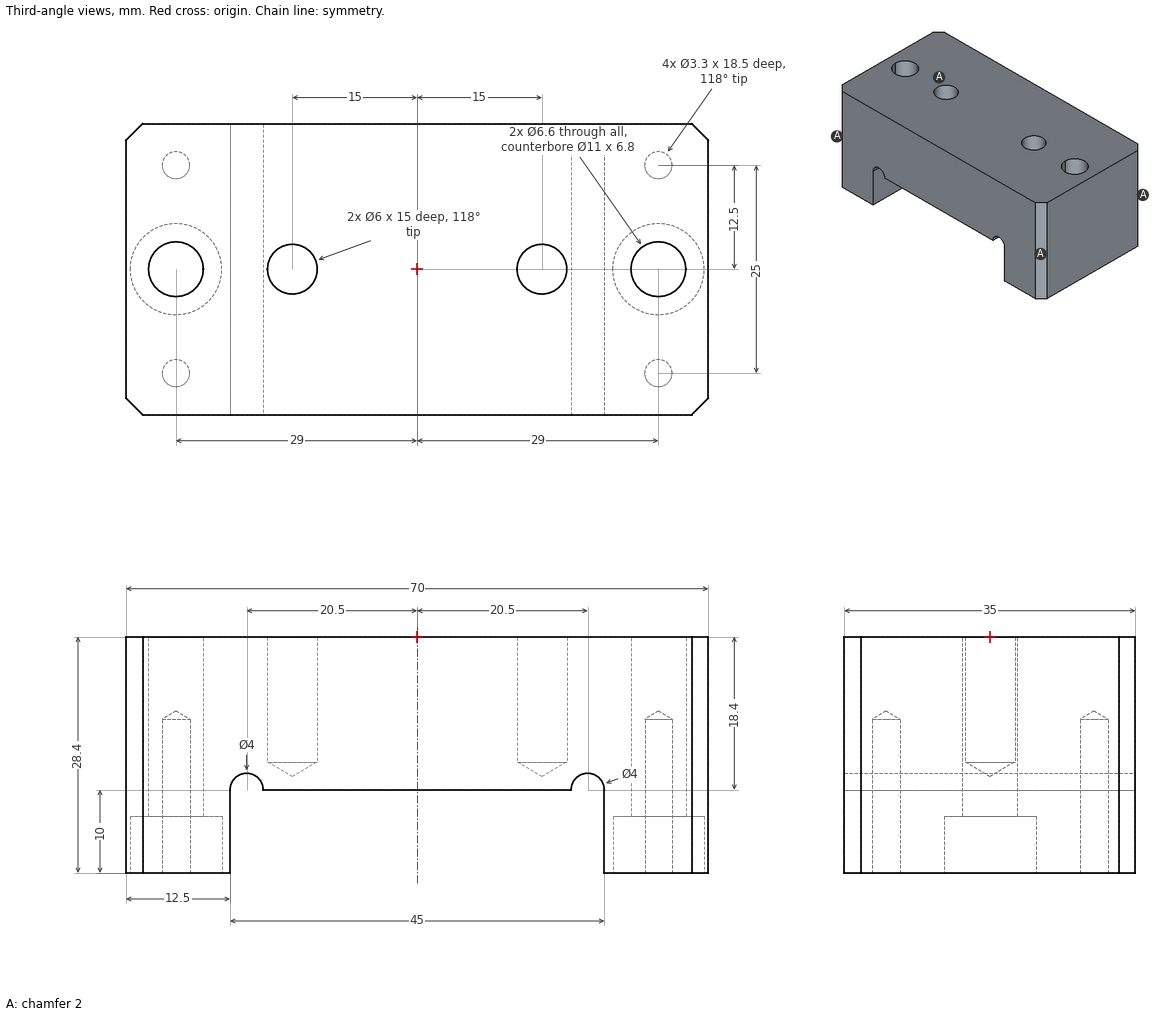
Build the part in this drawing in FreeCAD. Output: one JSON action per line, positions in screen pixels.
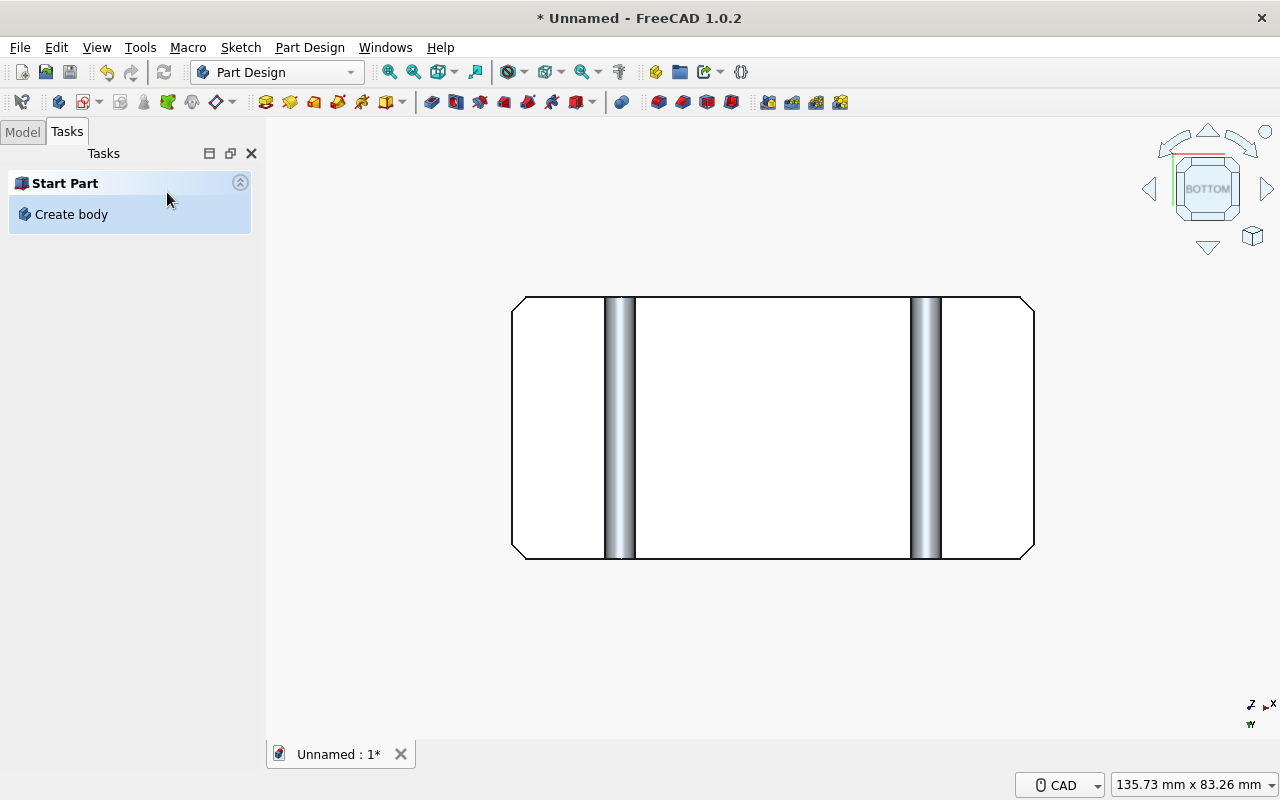
{"action": "left_click", "coordinate": [558, 502]}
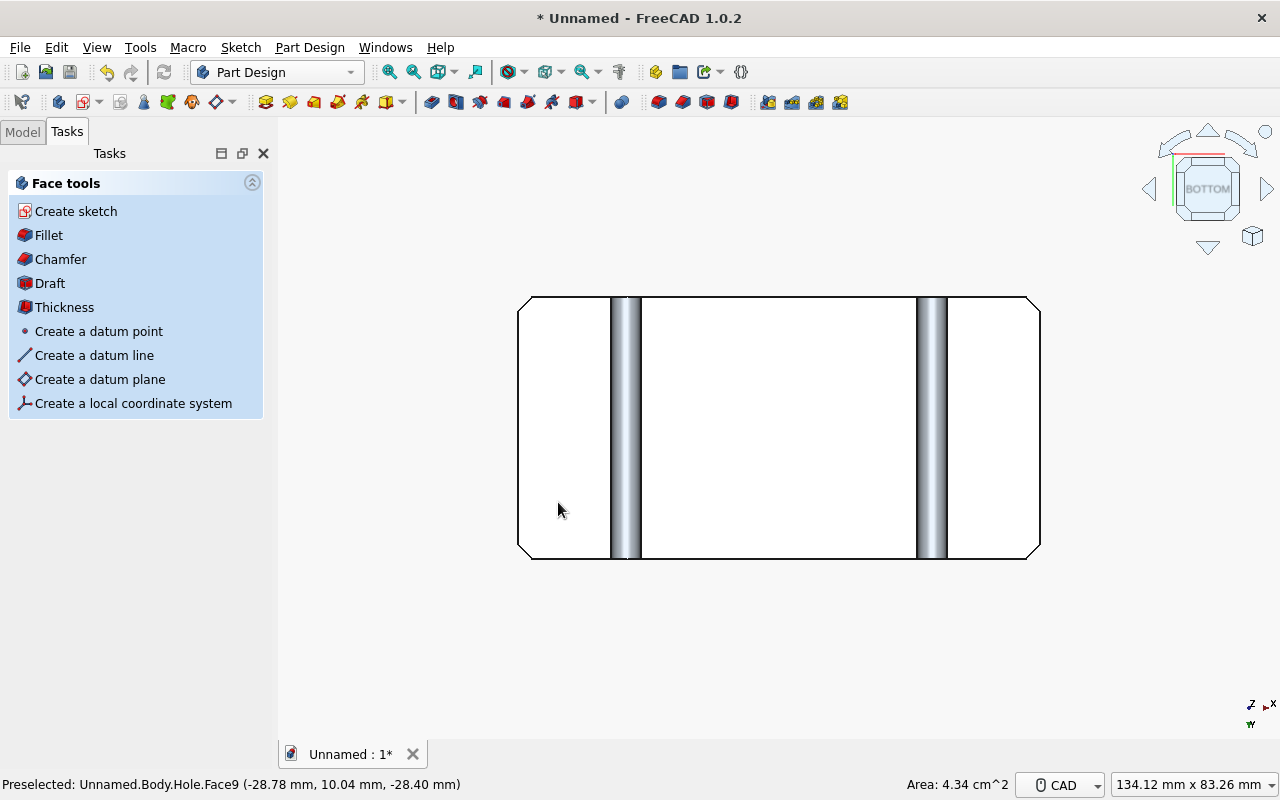
{"action": "left_click", "coordinate": [84, 102]}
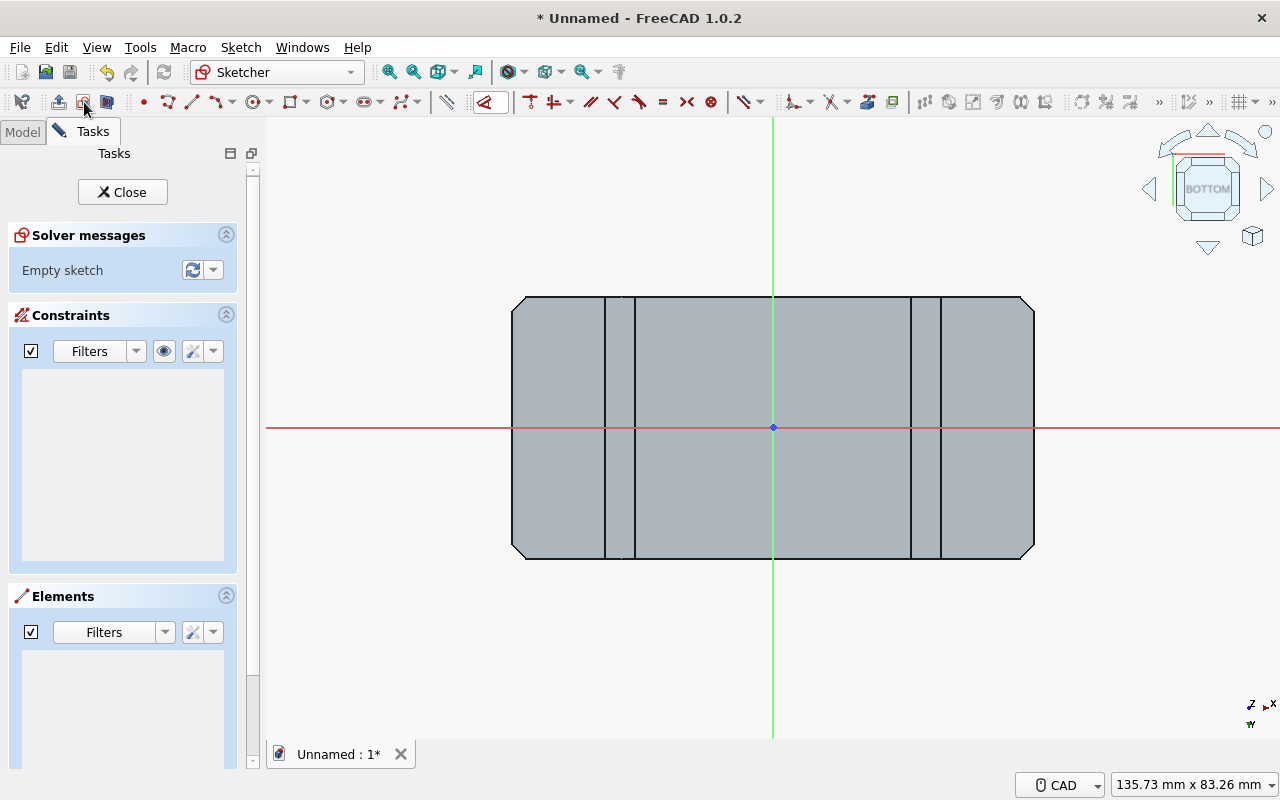
{"action": "left_click", "coordinate": [254, 102]}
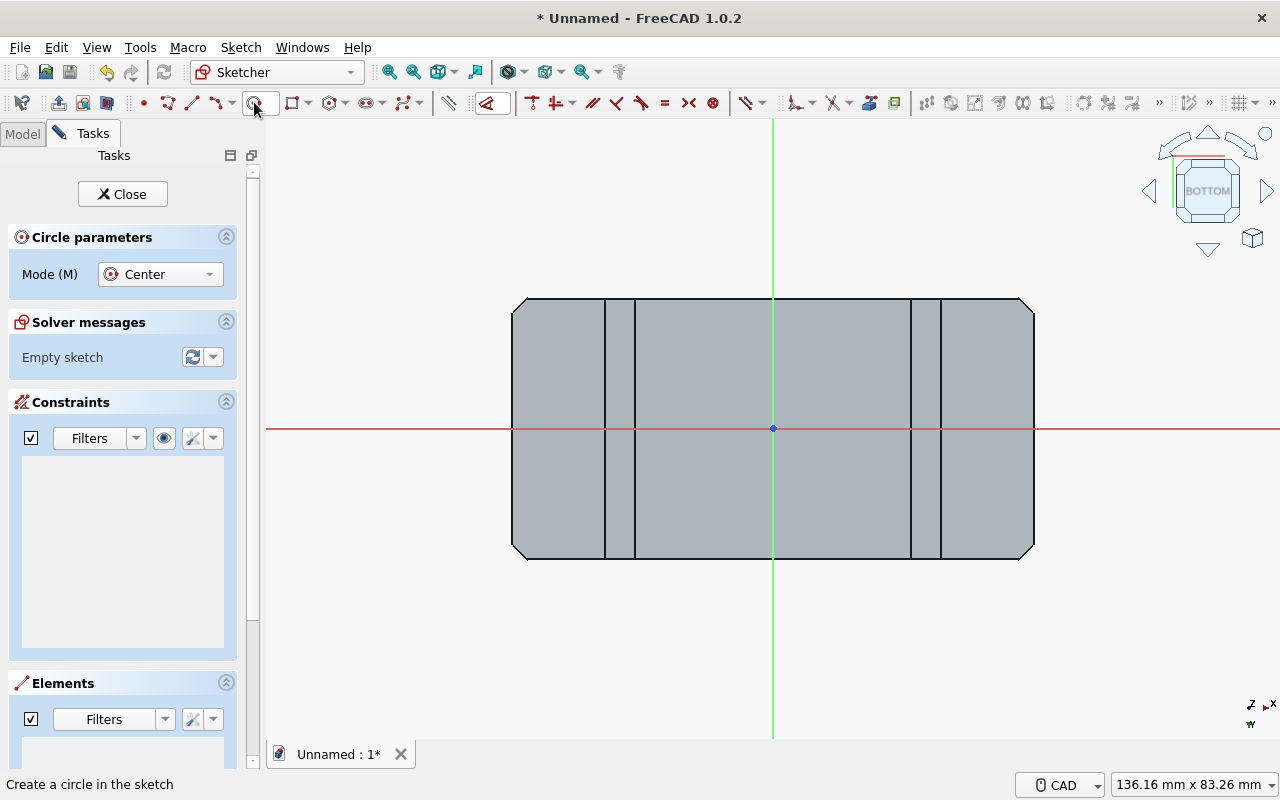
{"action": "left_click", "coordinate": [989, 429]}
{"action": "left_click", "coordinate": [1006, 412]}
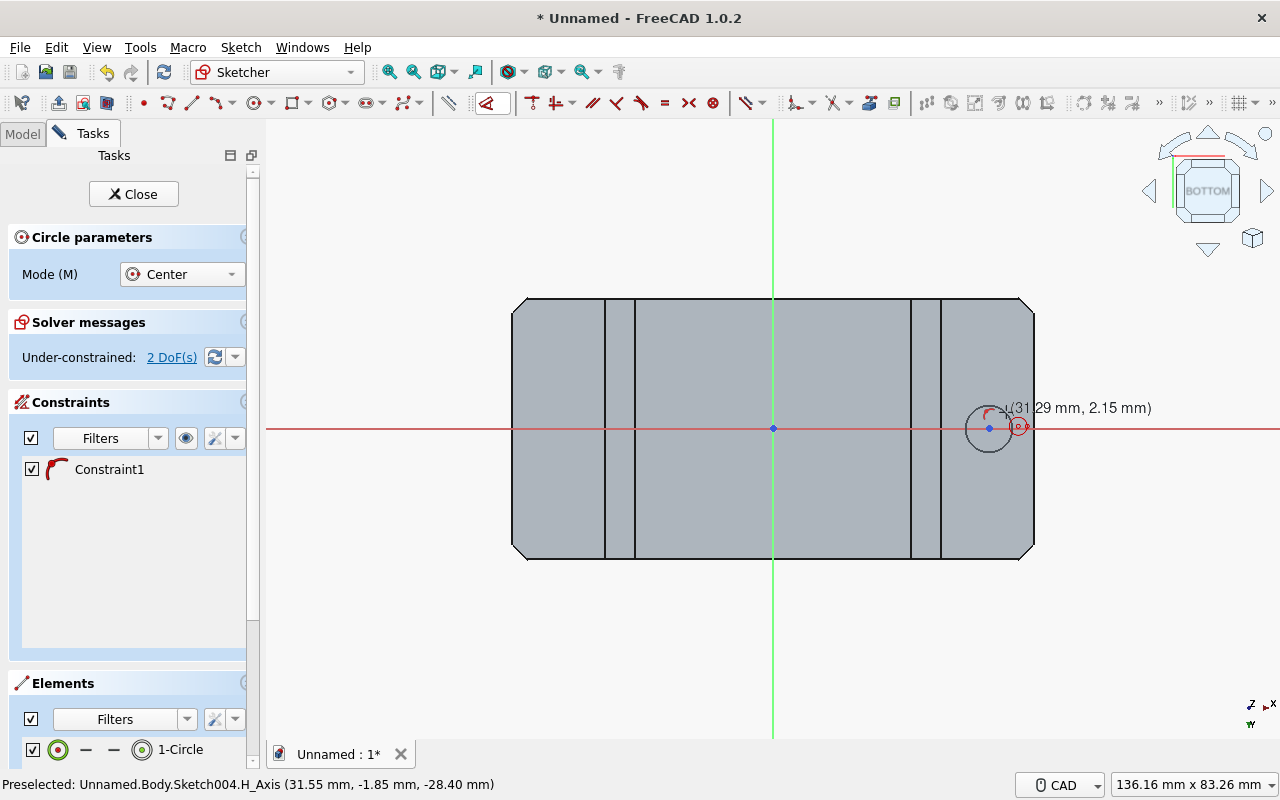
{"action": "left_click", "coordinate": [557, 429]}
{"action": "left_click", "coordinate": [574, 412]}
{"action": "key", "text": "Escape"}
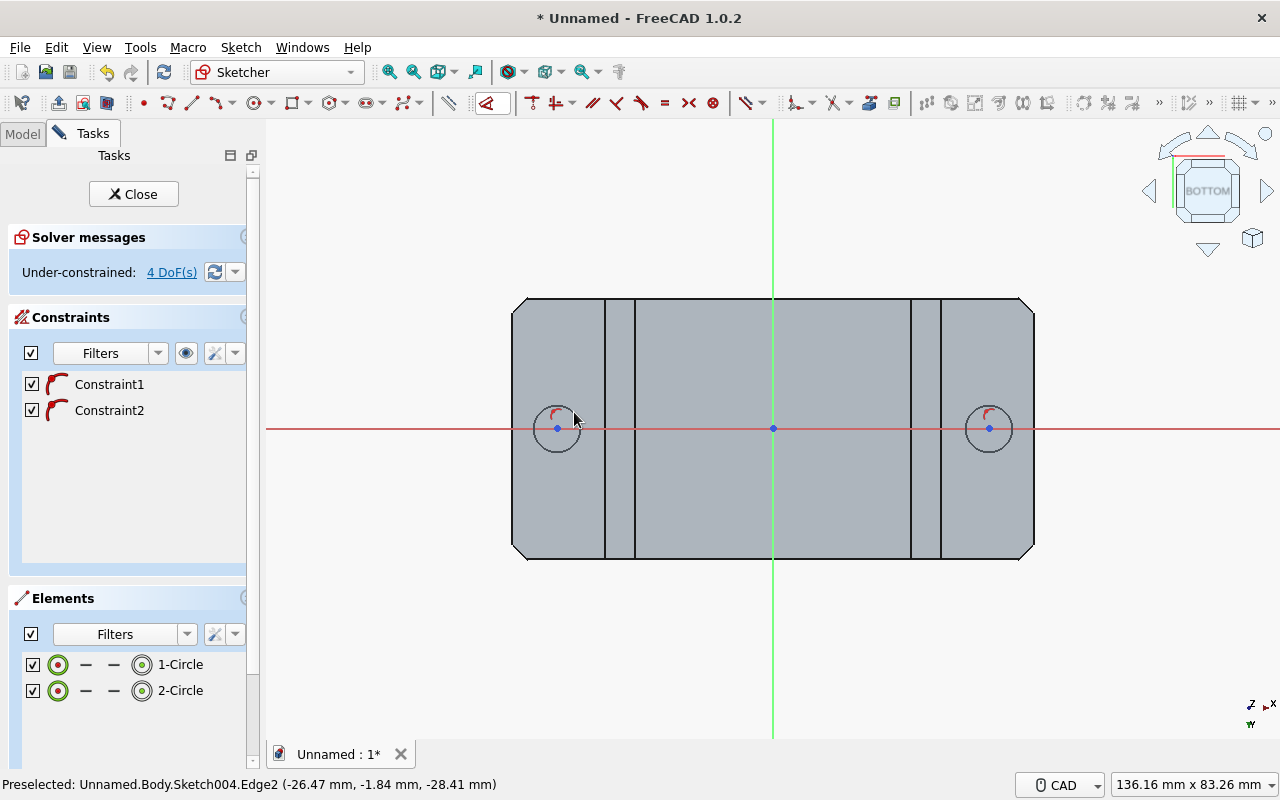
{"action": "left_click", "coordinate": [1005, 412]}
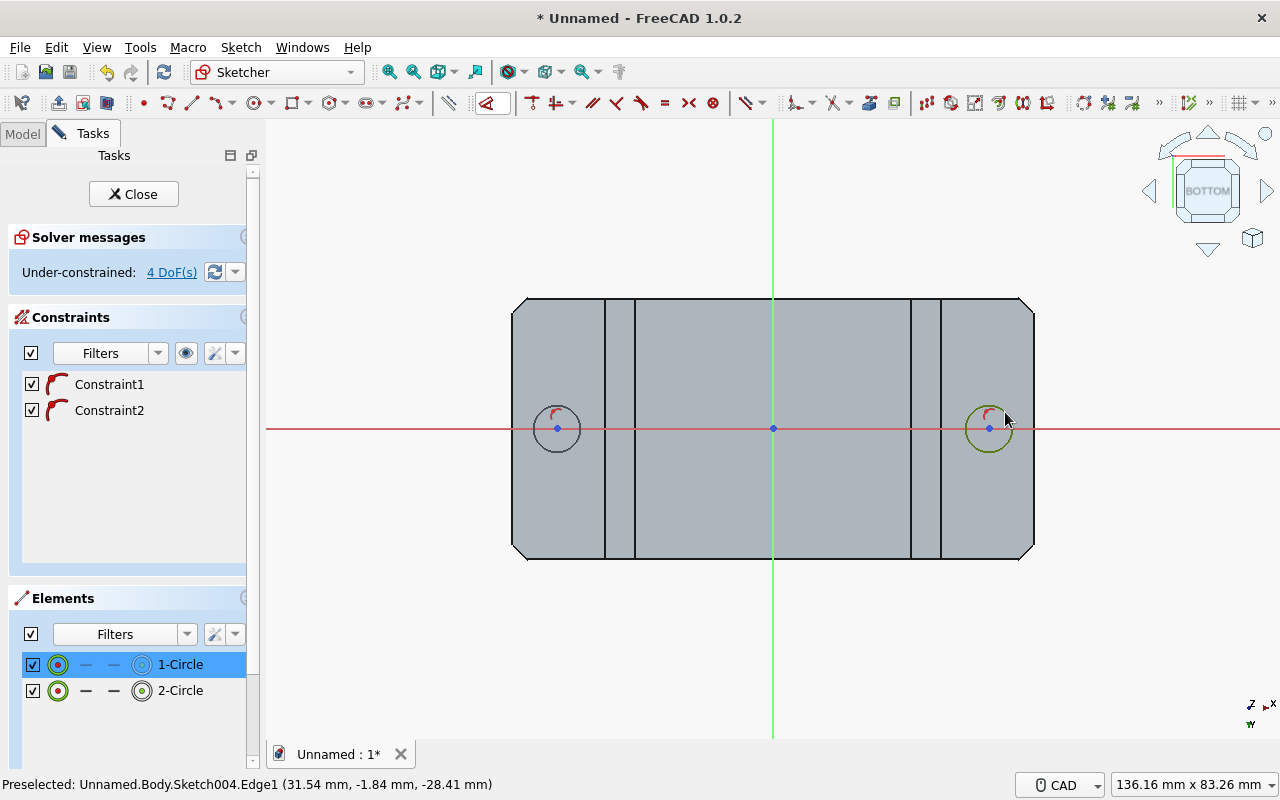
{"action": "left_click", "coordinate": [573, 412]}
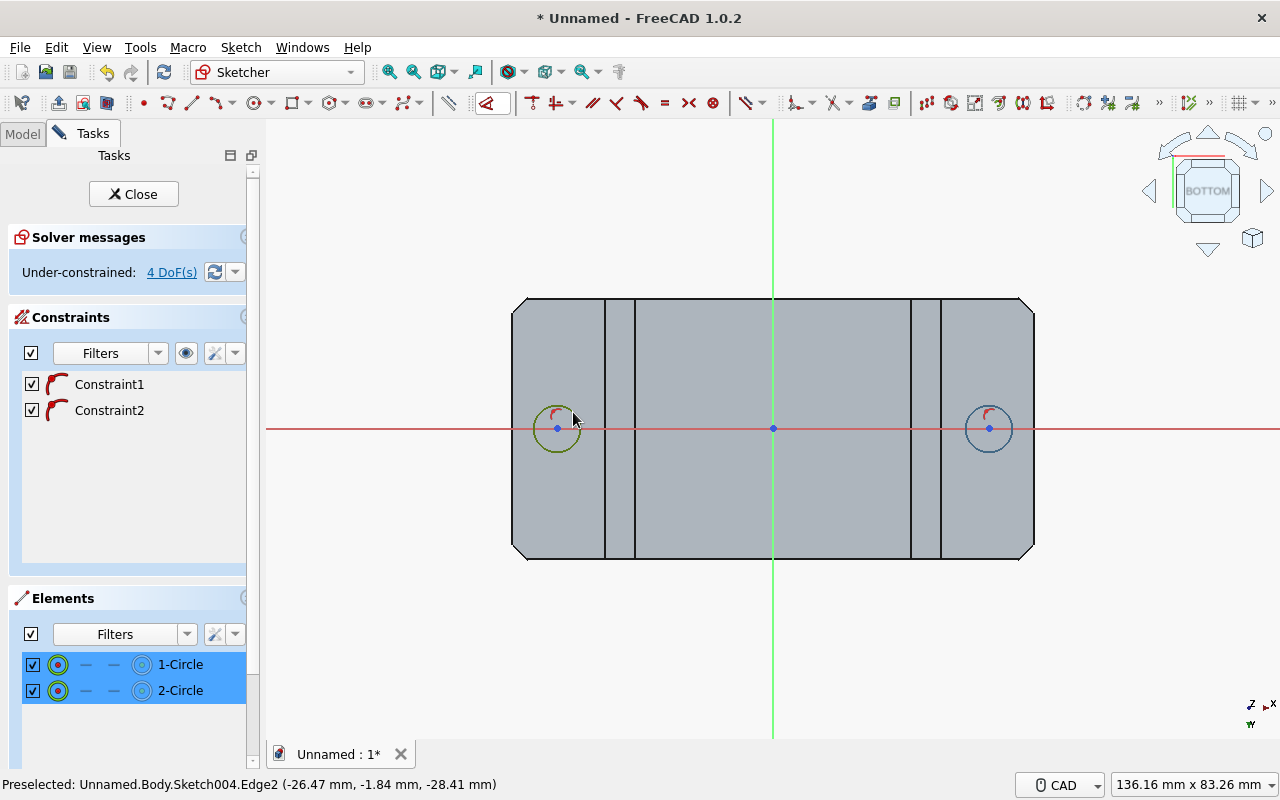
{"action": "left_click", "coordinate": [666, 104]}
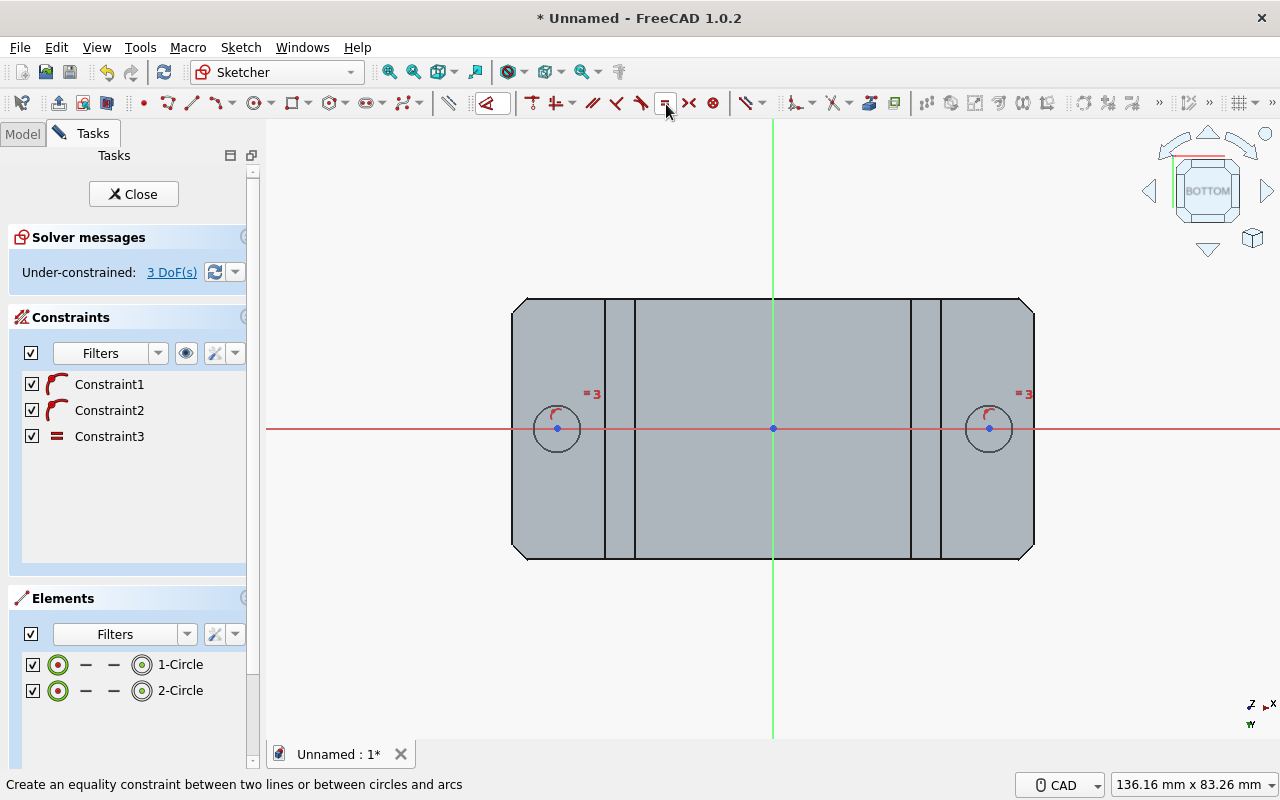
{"action": "key", "text": "d"}